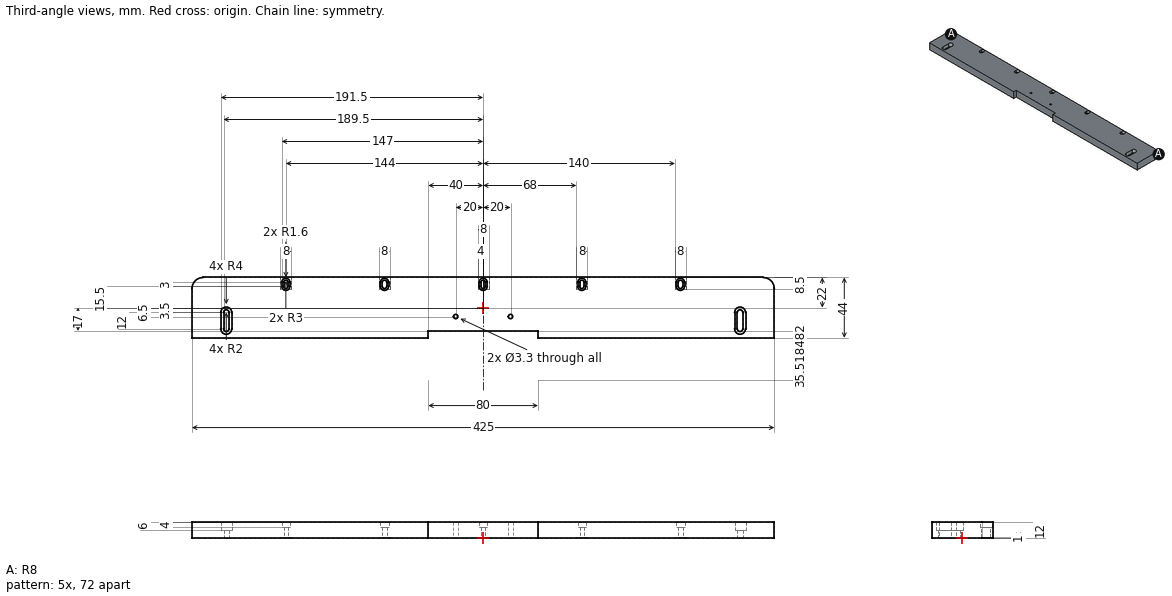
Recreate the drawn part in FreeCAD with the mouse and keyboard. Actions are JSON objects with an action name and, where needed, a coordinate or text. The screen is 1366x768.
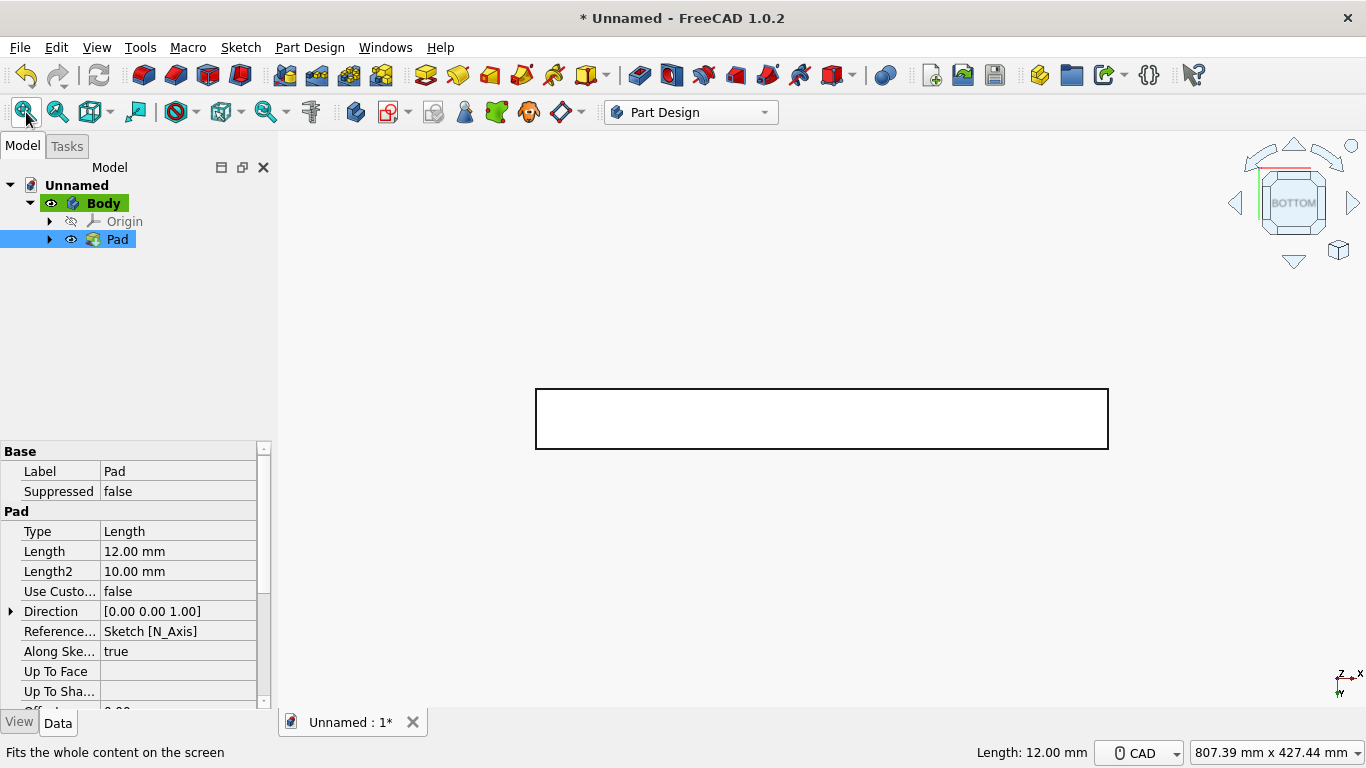
{"action": "scroll", "coordinate": [536, 448], "scroll_direction": "up", "scroll_amount": 5}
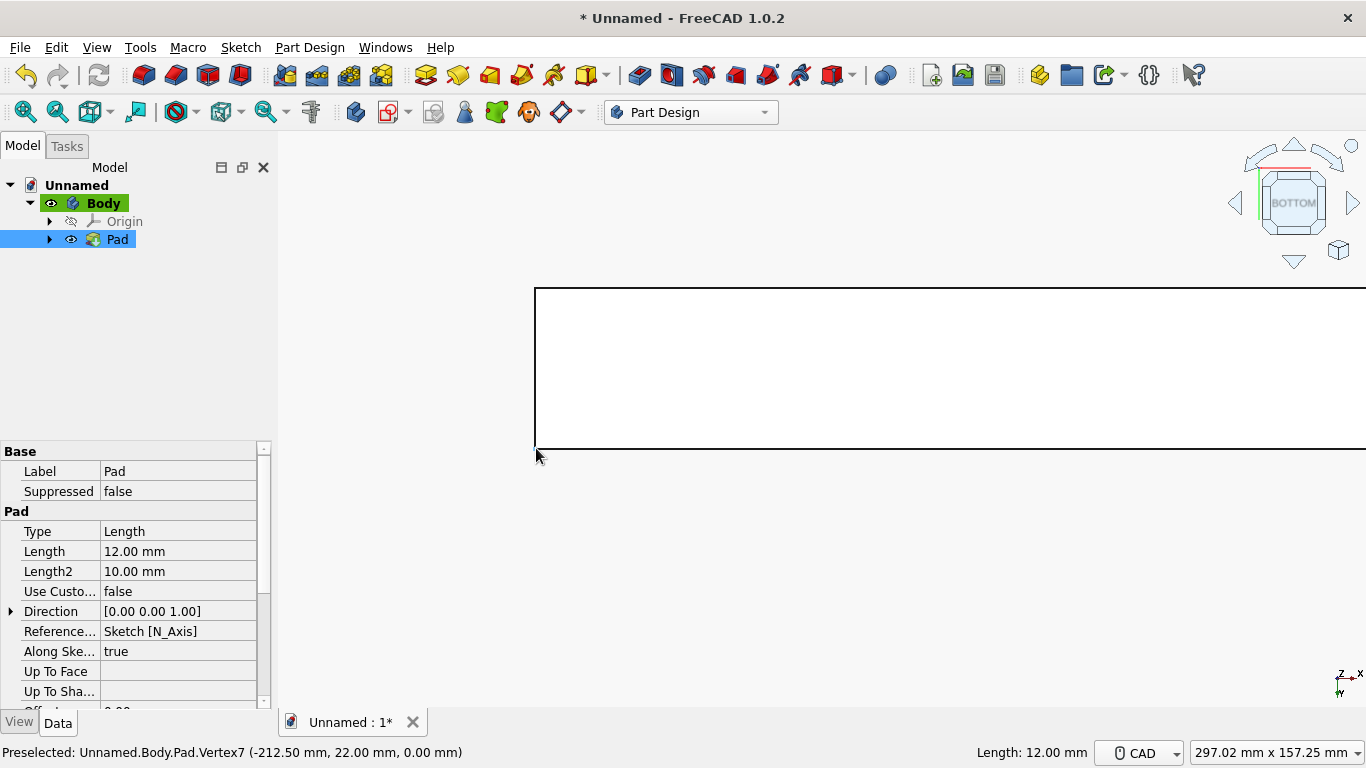
{"action": "left_click", "coordinate": [26, 112]}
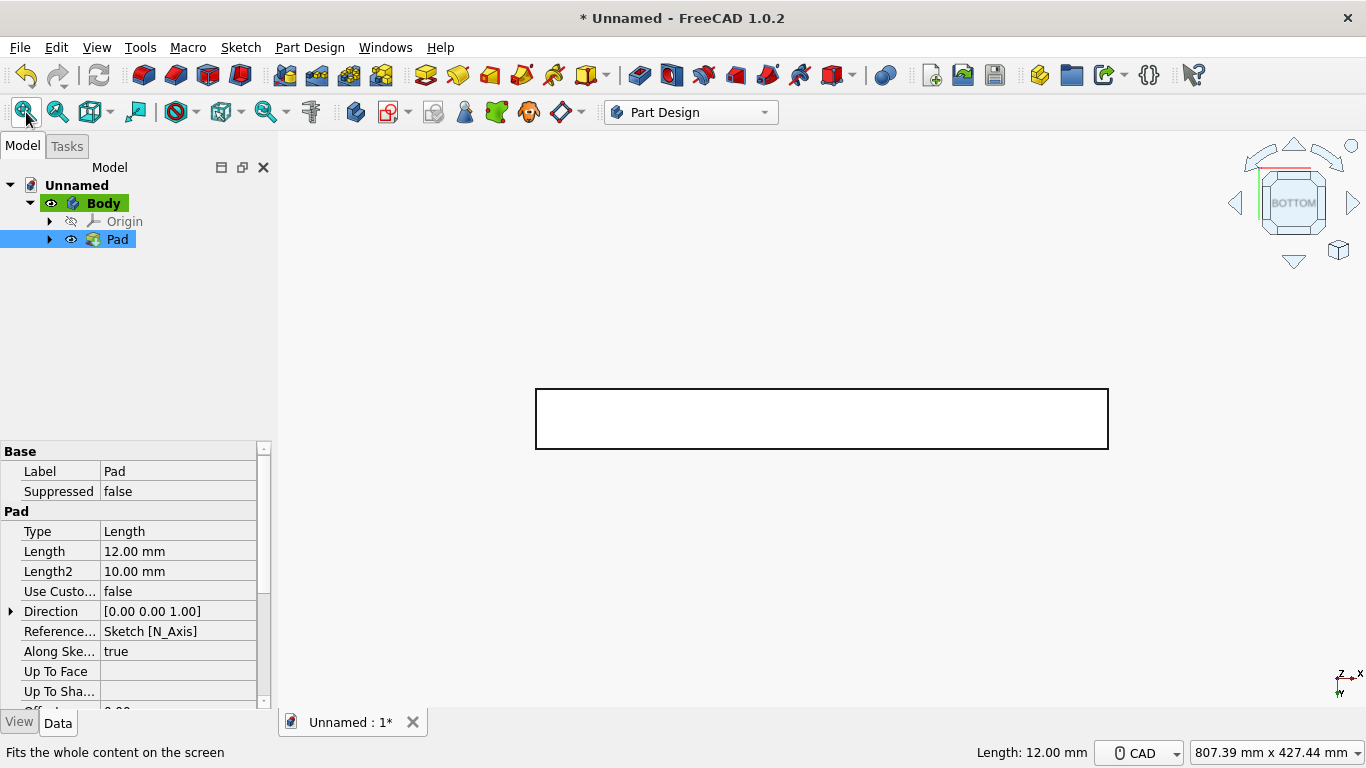
{"action": "key", "text": "4"}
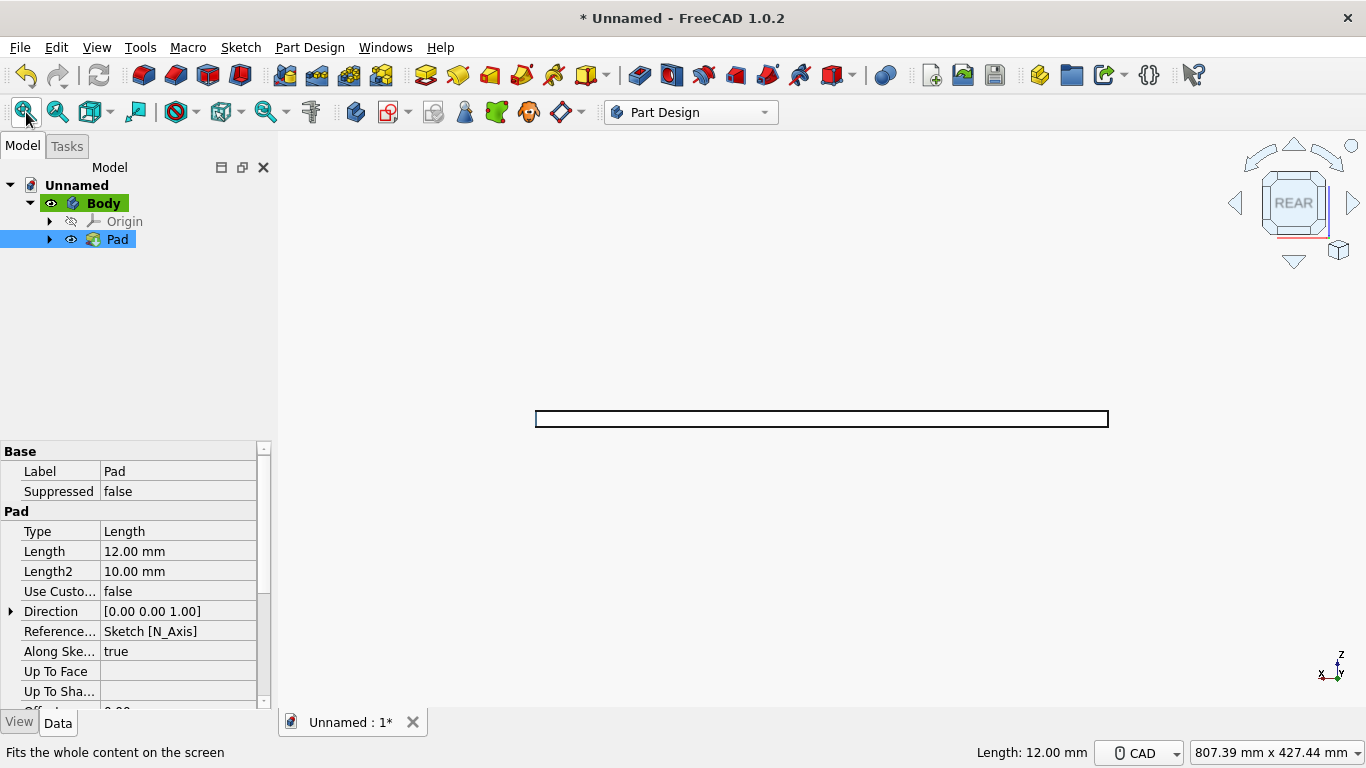
{"action": "left_click", "coordinate": [1108, 418], "text": "ctrl"}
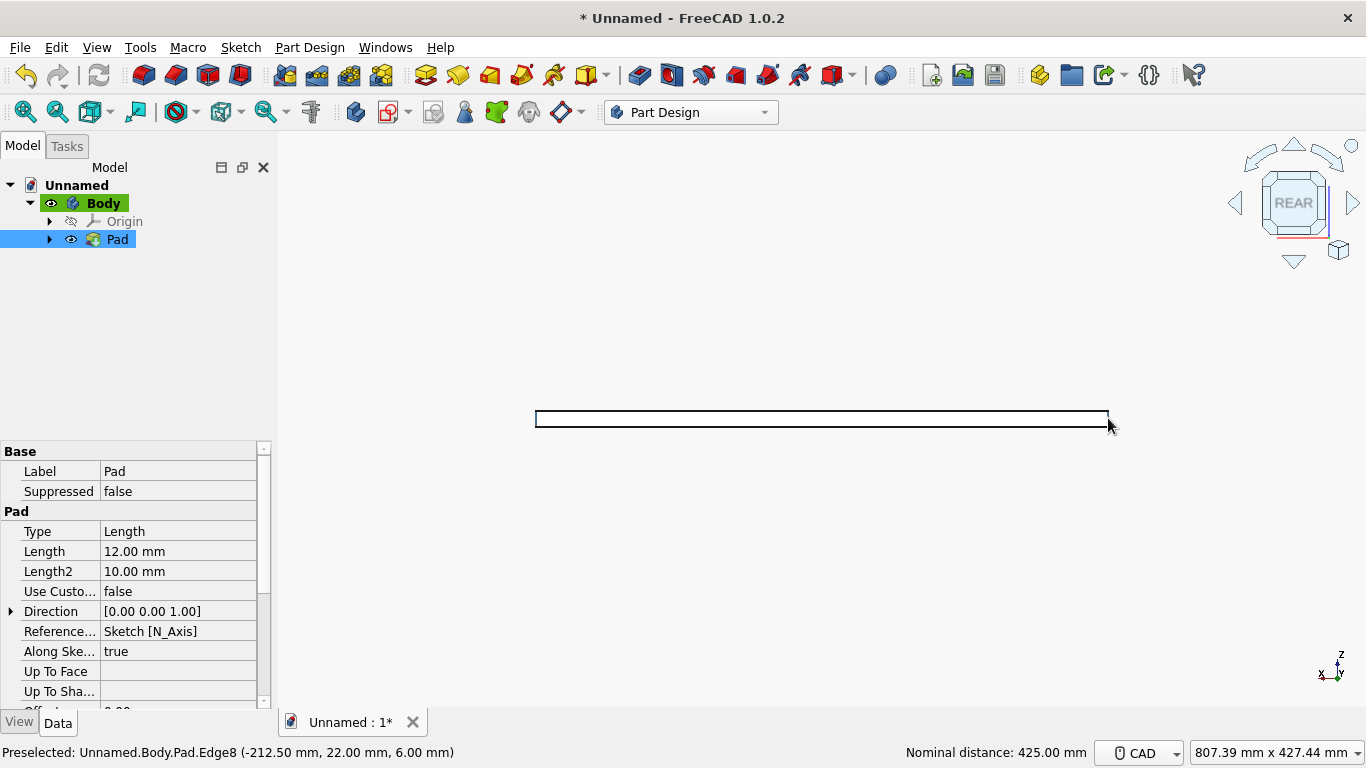
{"action": "left_click", "coordinate": [144, 76]}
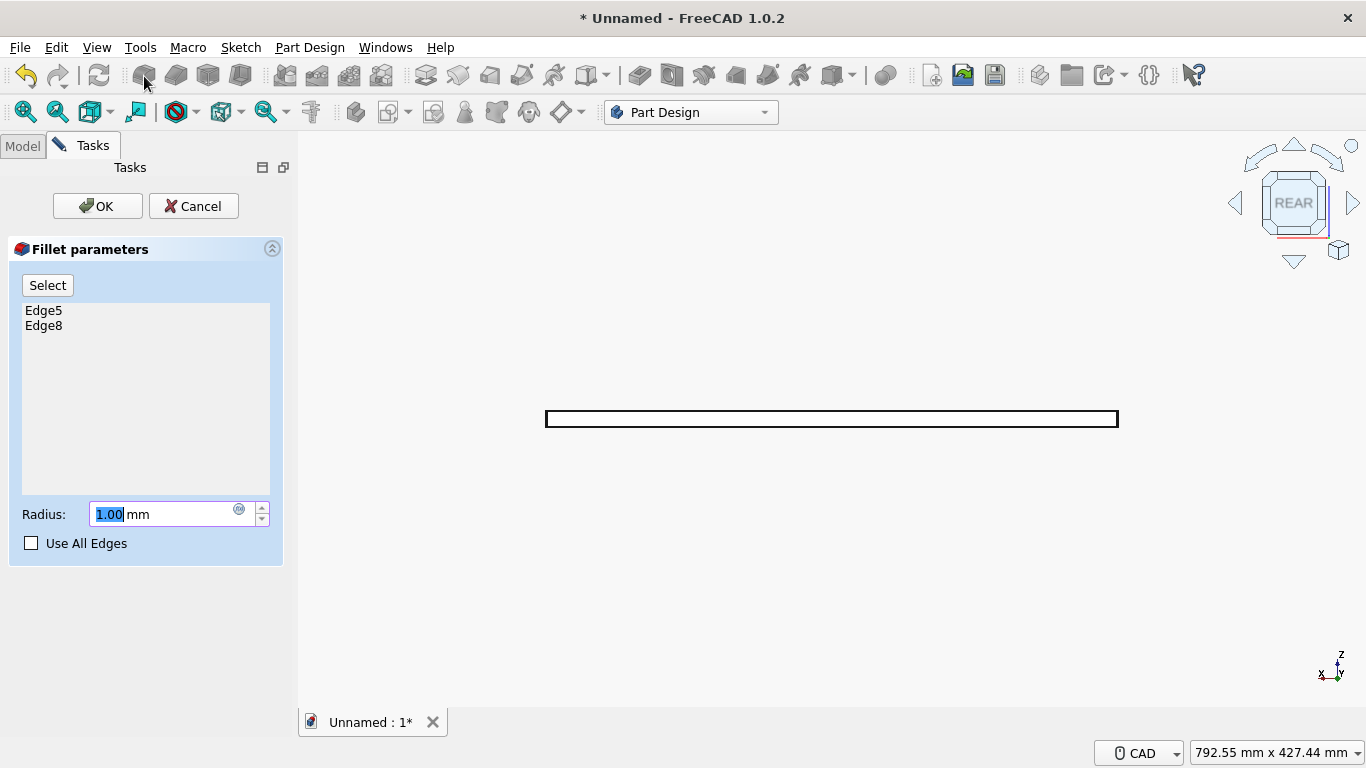
{"action": "type", "text": "8"}
{"action": "key", "text": "Tab"}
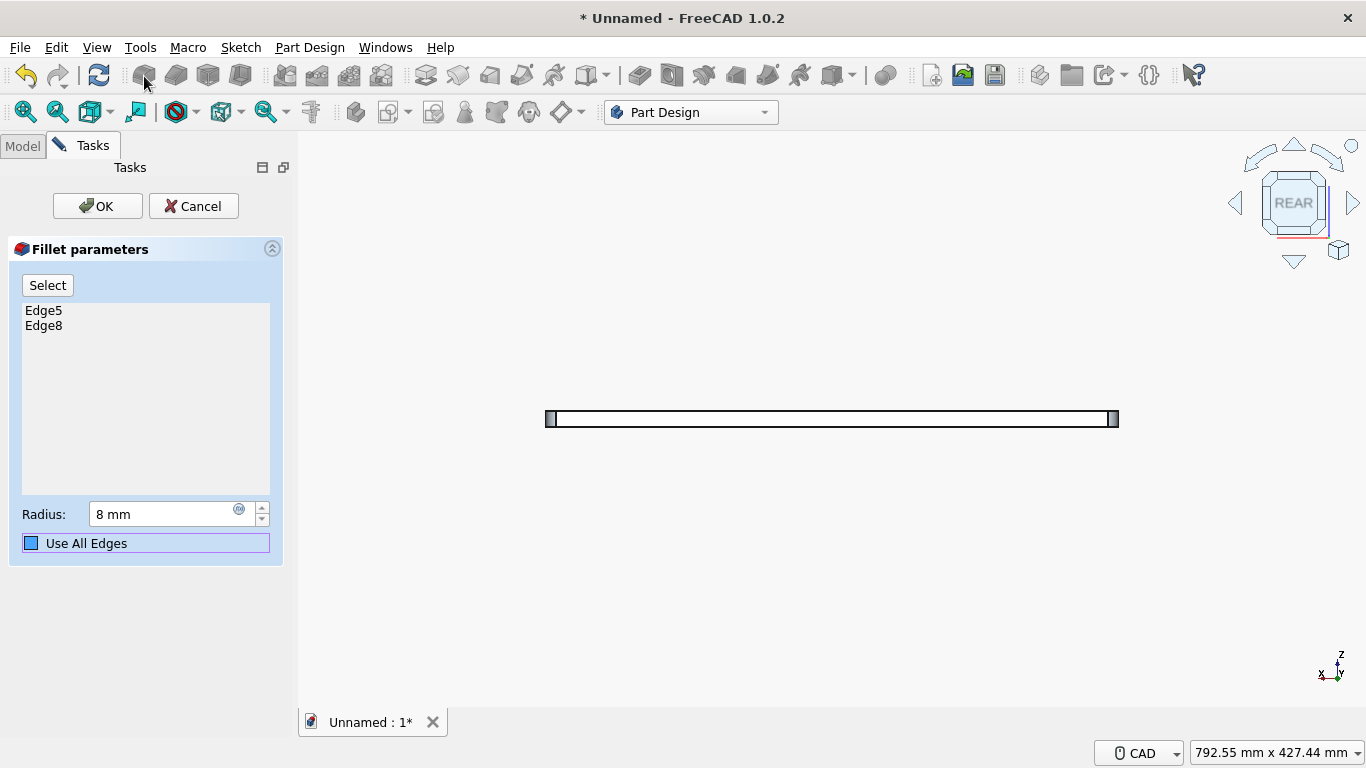
{"action": "left_click", "coordinate": [98, 206]}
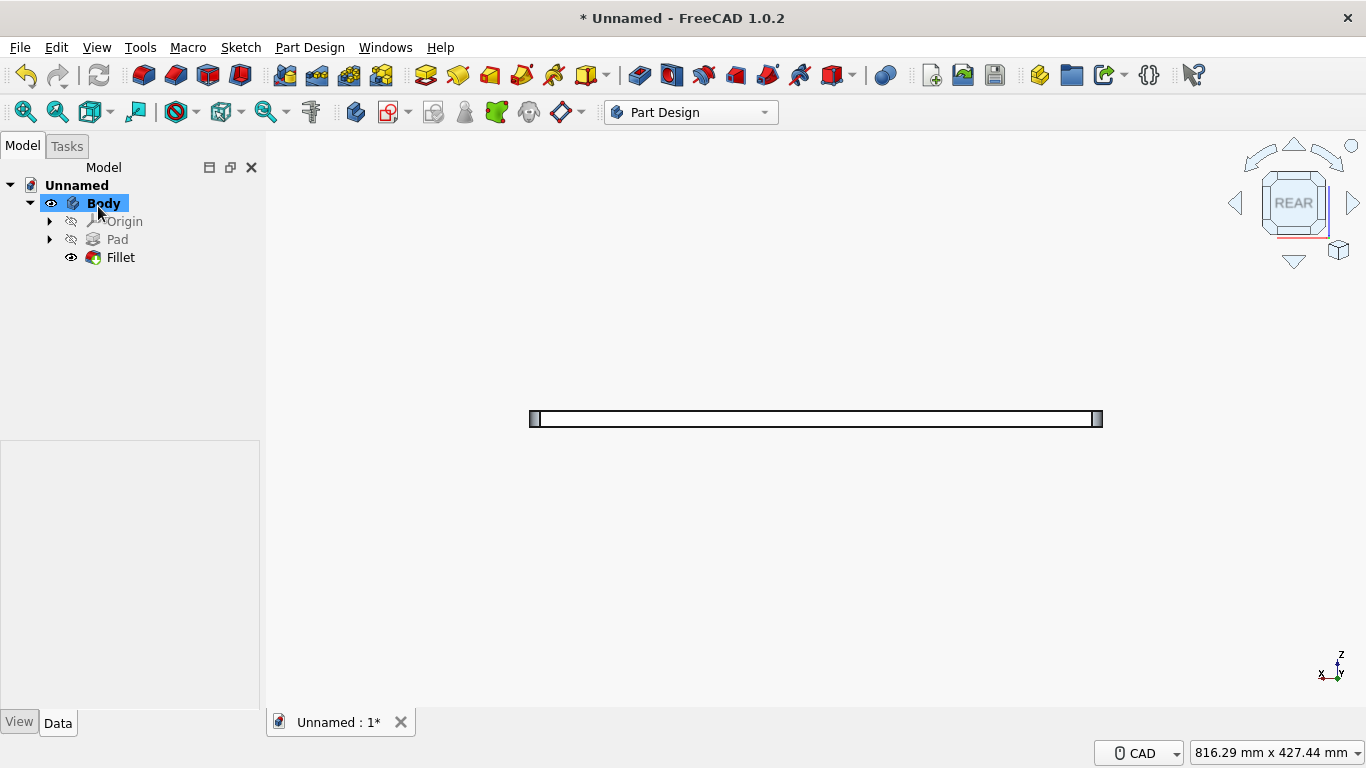
{"action": "key", "text": "0"}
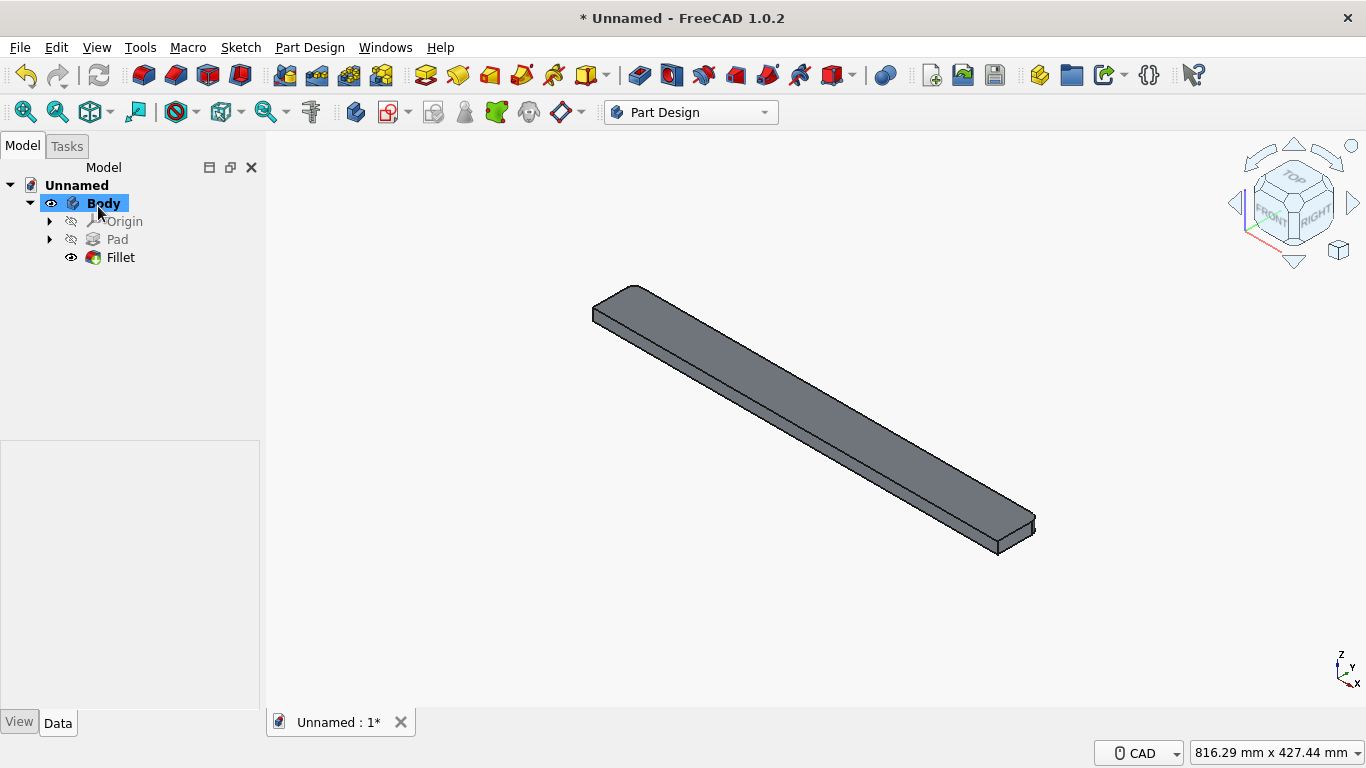
{"action": "left_click", "coordinate": [990, 512]}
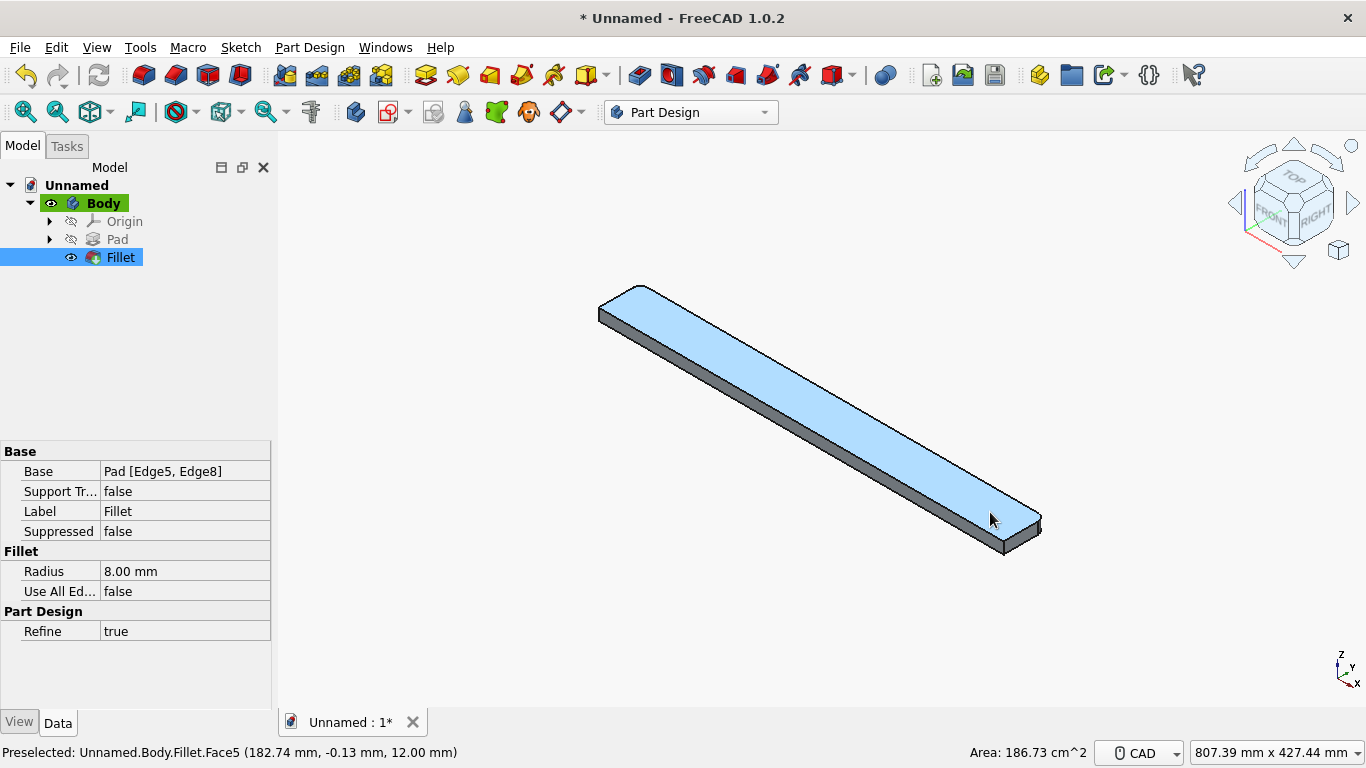
{"action": "left_click", "coordinate": [388, 112]}